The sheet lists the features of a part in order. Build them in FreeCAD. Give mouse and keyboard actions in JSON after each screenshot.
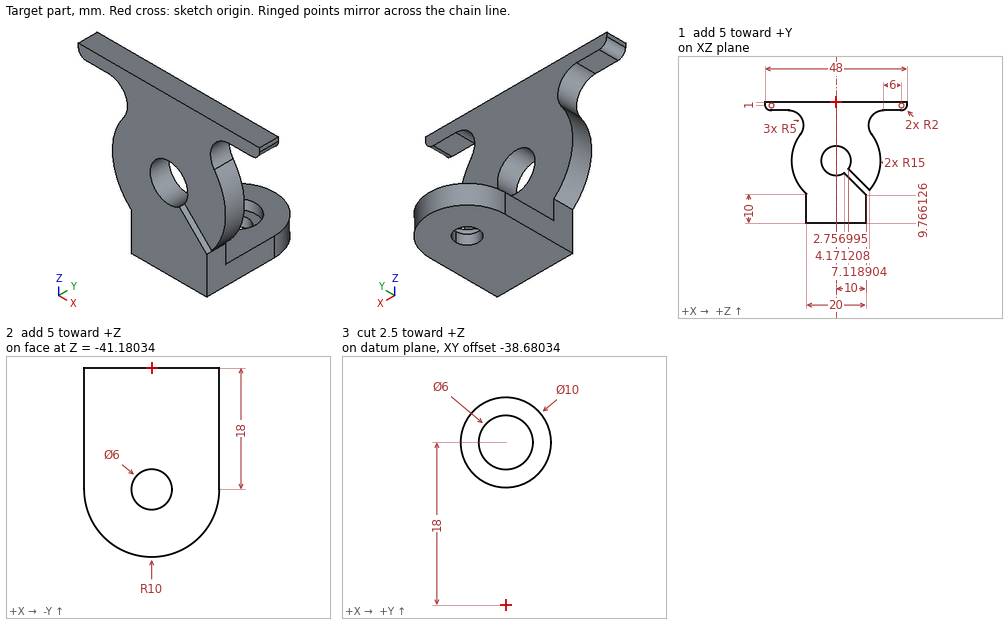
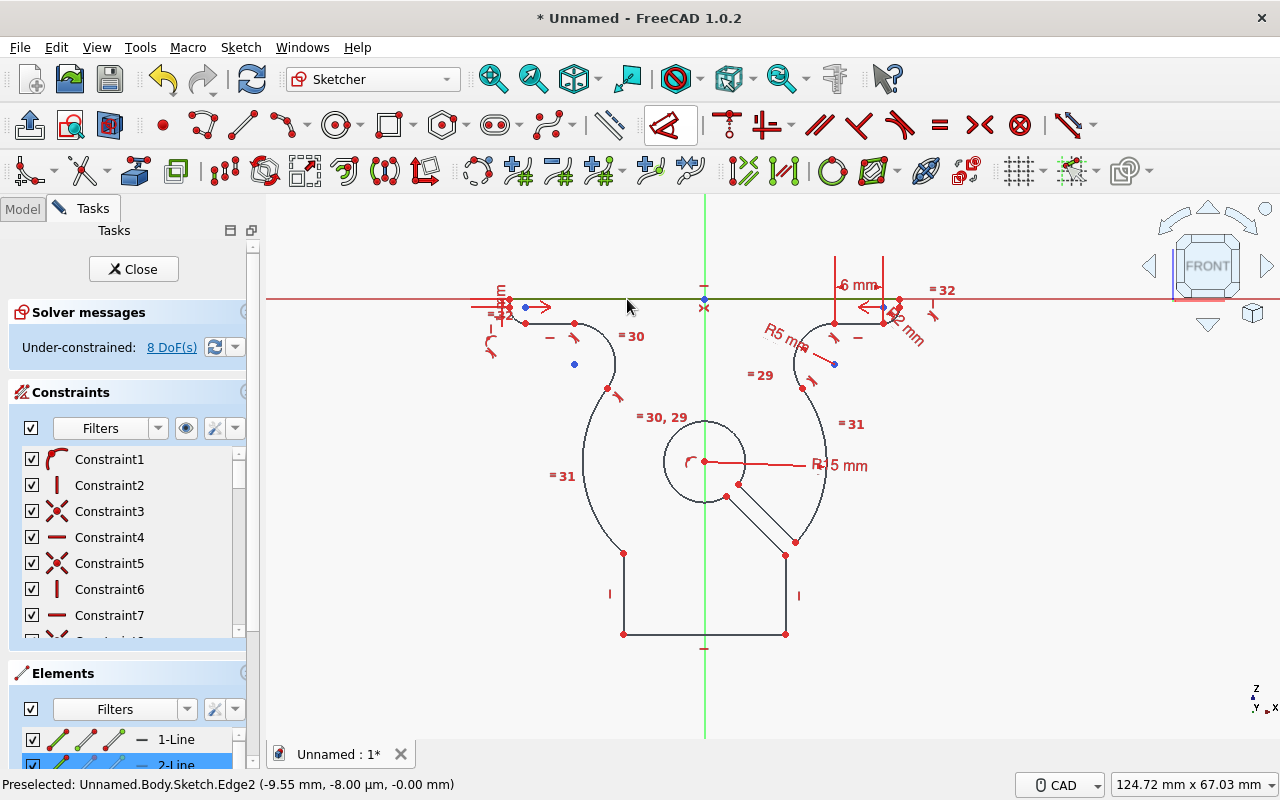
{"action": "key", "text": "l"}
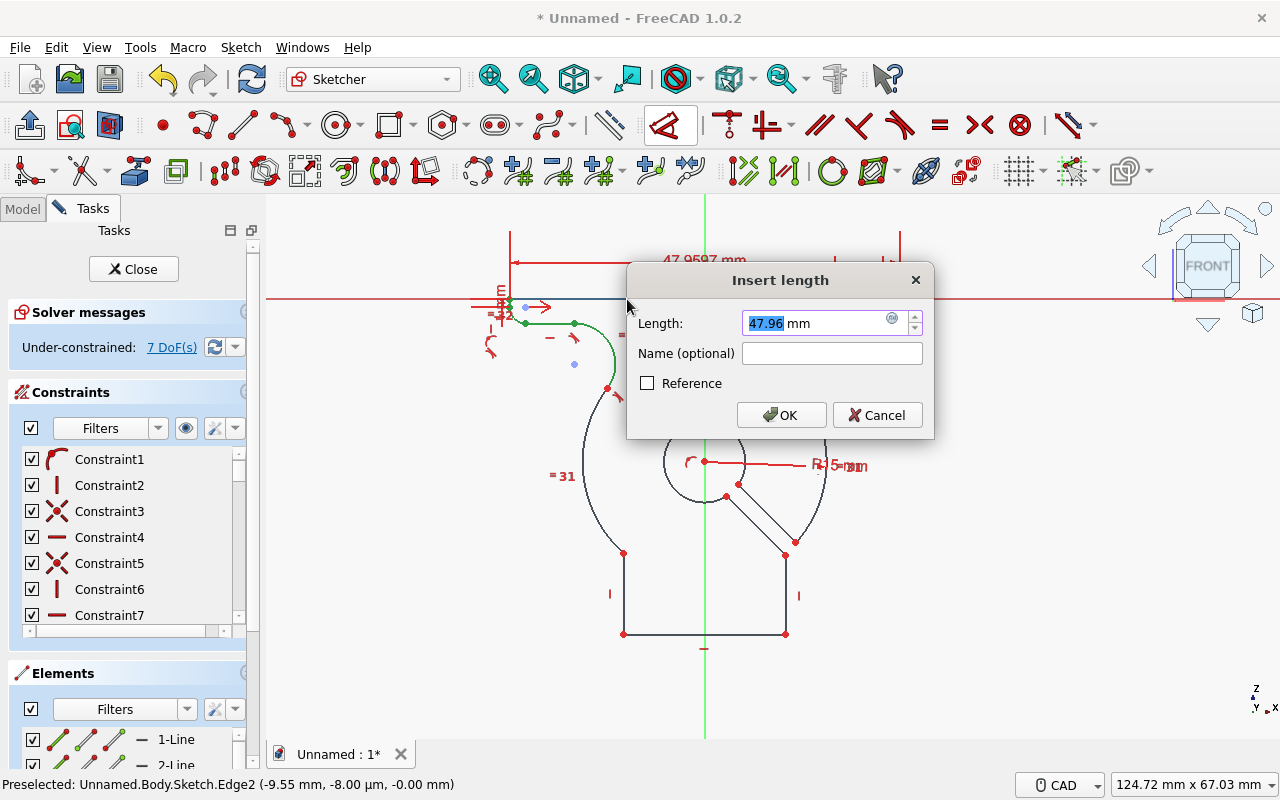
{"action": "type", "text": "48"}
{"action": "key", "text": "Return"}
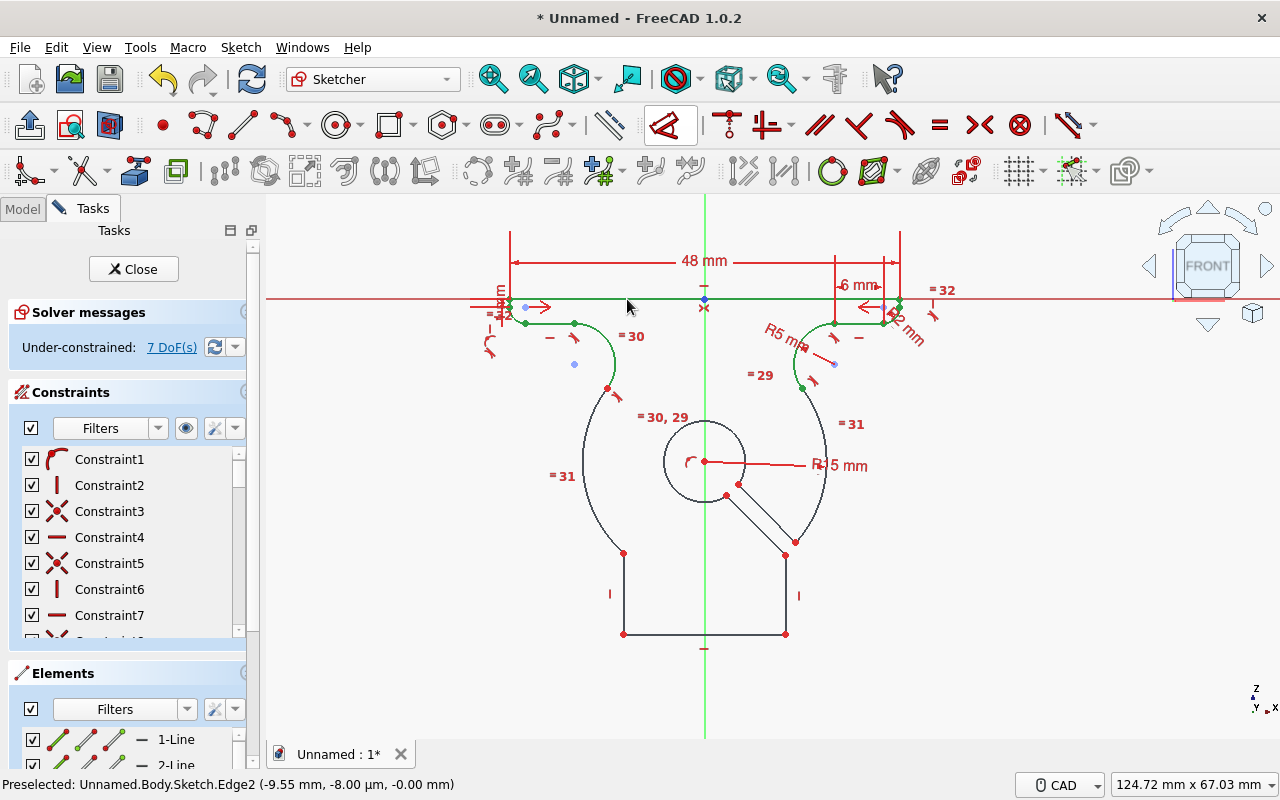
{"action": "left_click", "coordinate": [737, 635]}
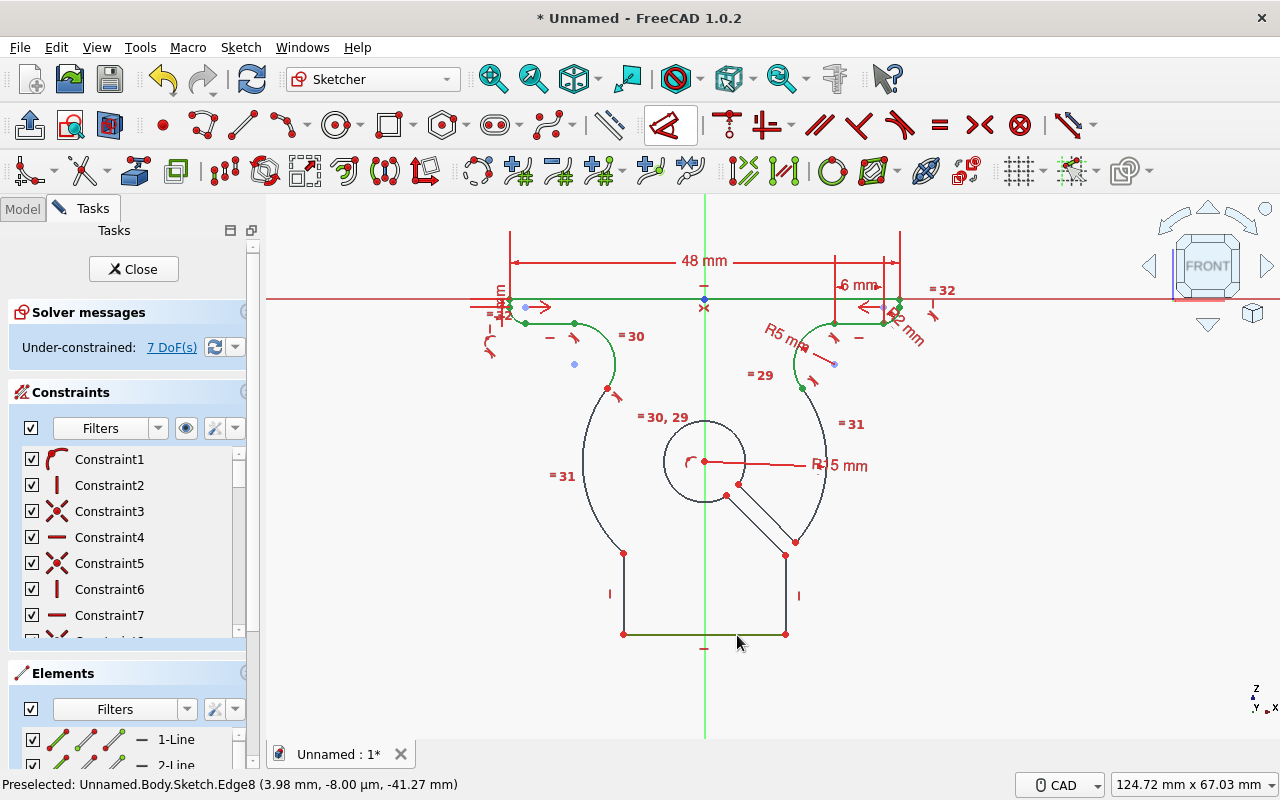
{"action": "key", "text": "l"}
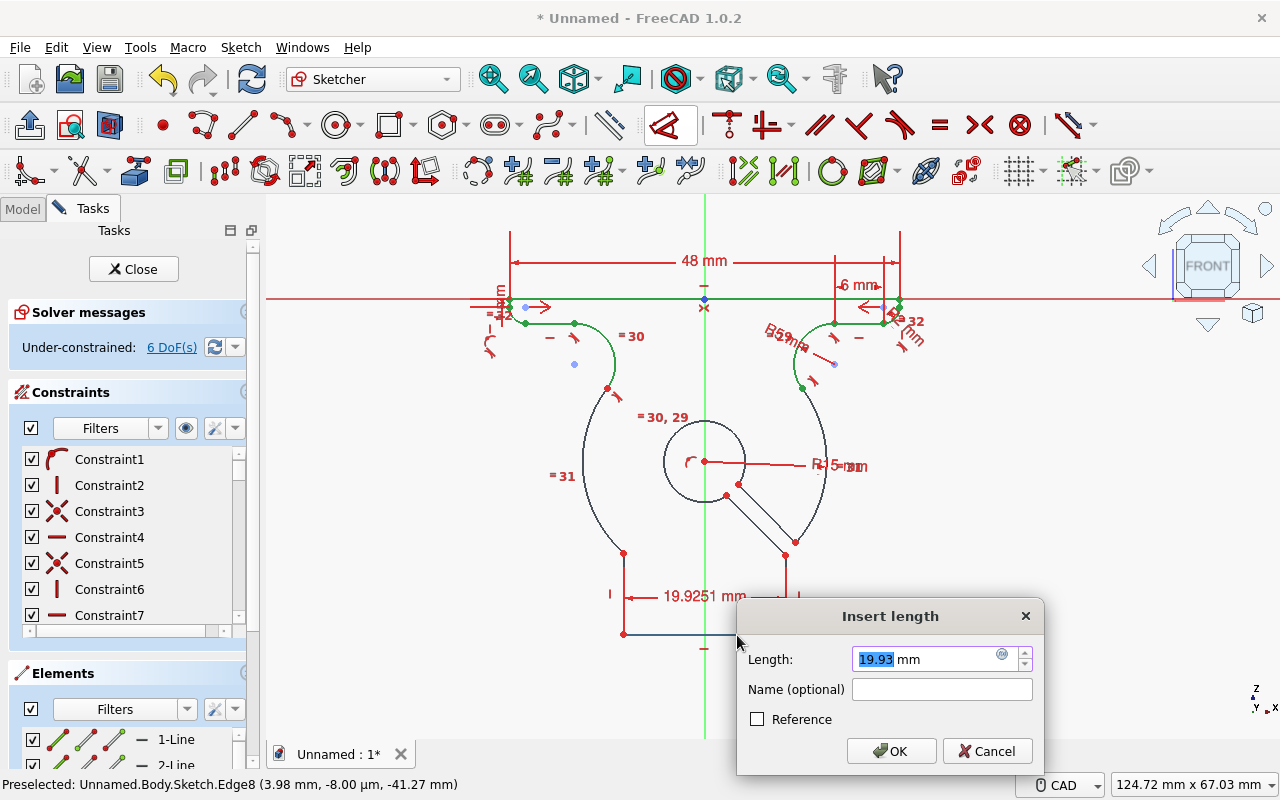
{"action": "type", "text": "20"}
{"action": "key", "text": "Return"}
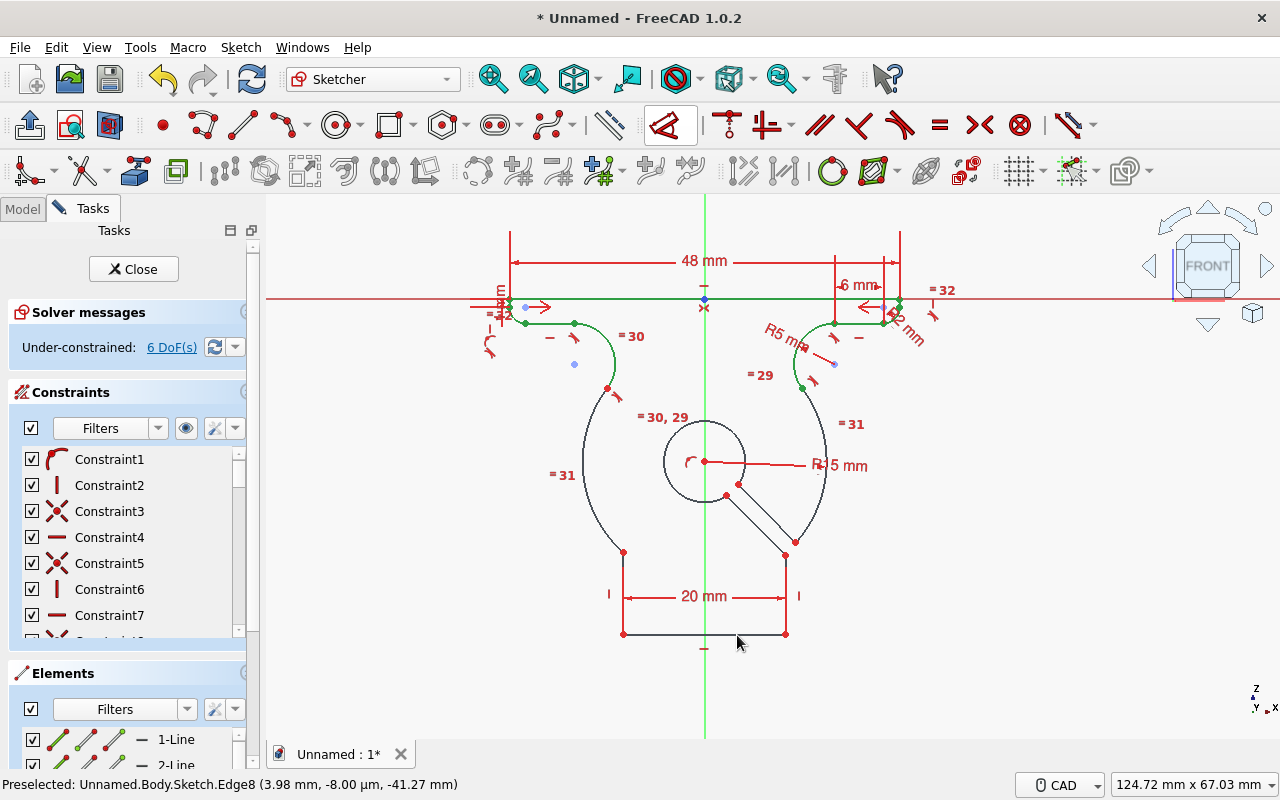
{"action": "left_click", "coordinate": [623, 610]}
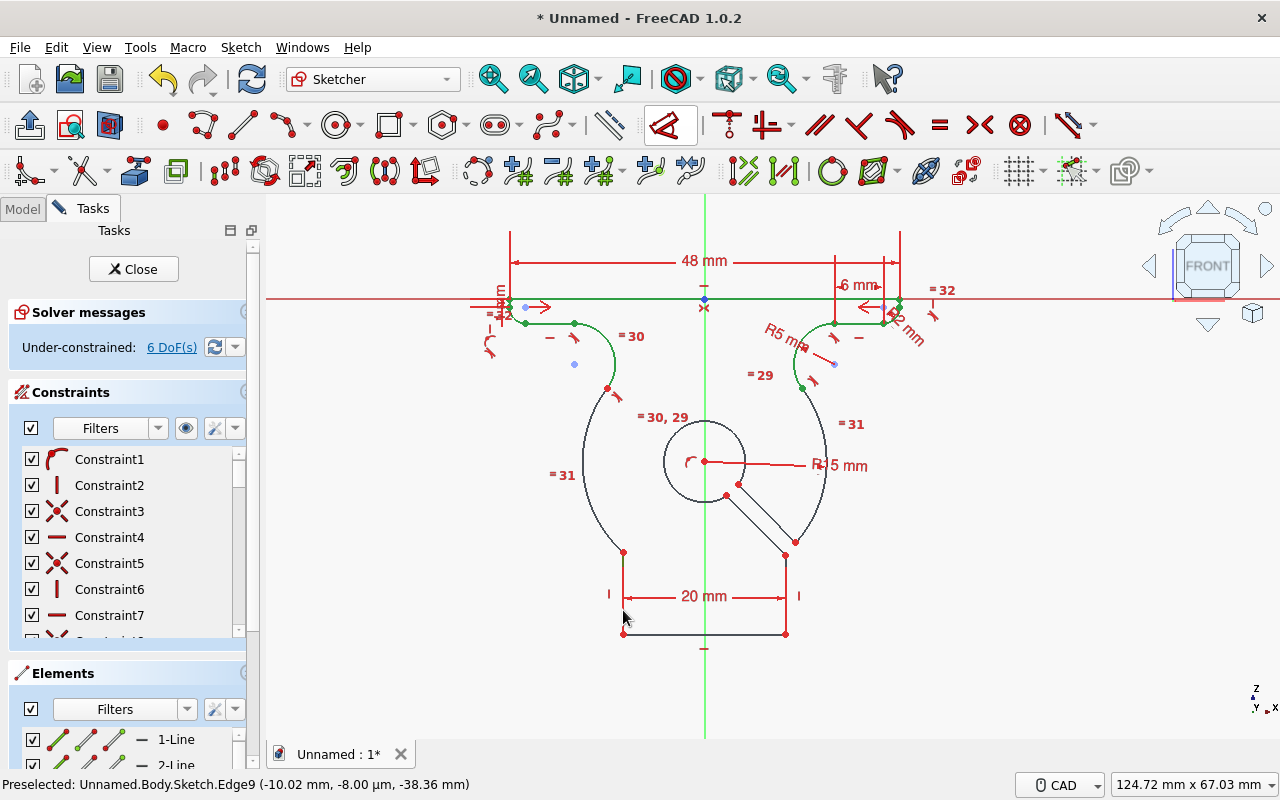
{"action": "key", "text": "i"}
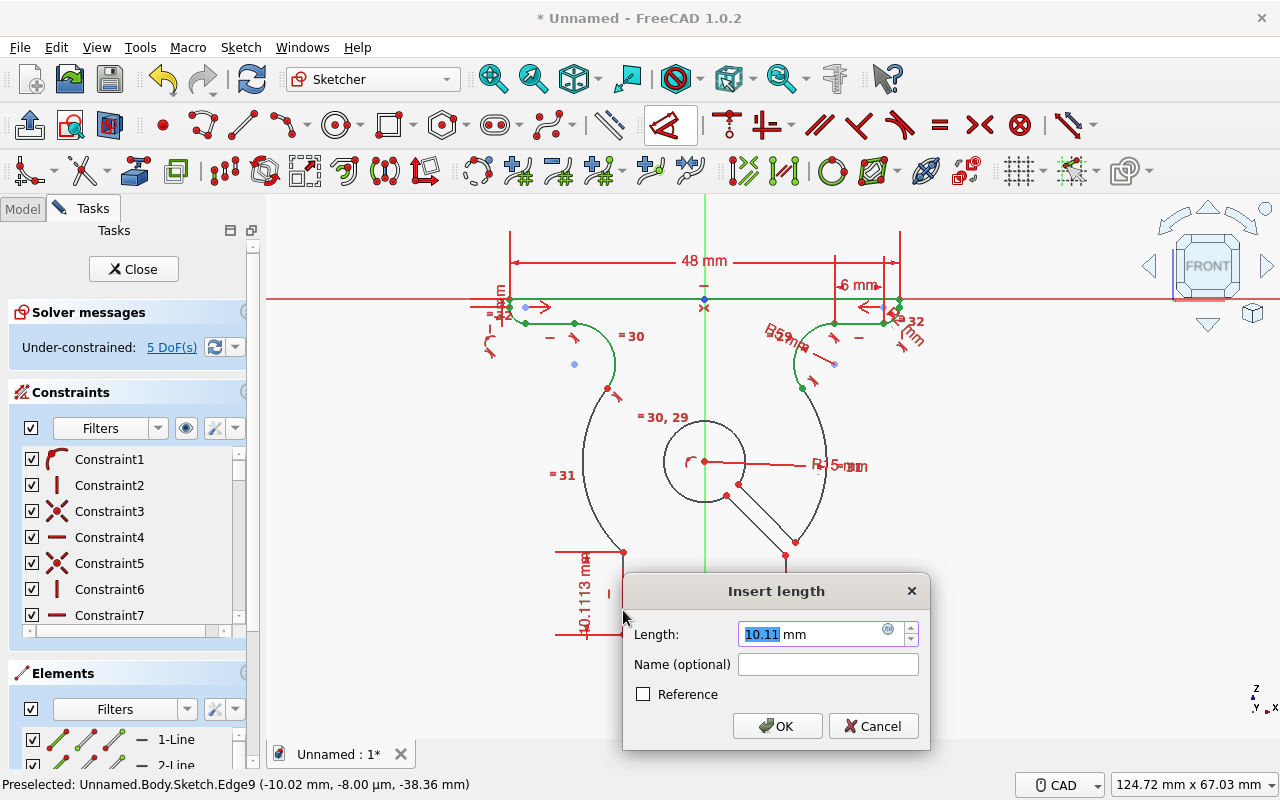
{"action": "type", "text": "10"}
{"action": "key", "text": "Return"}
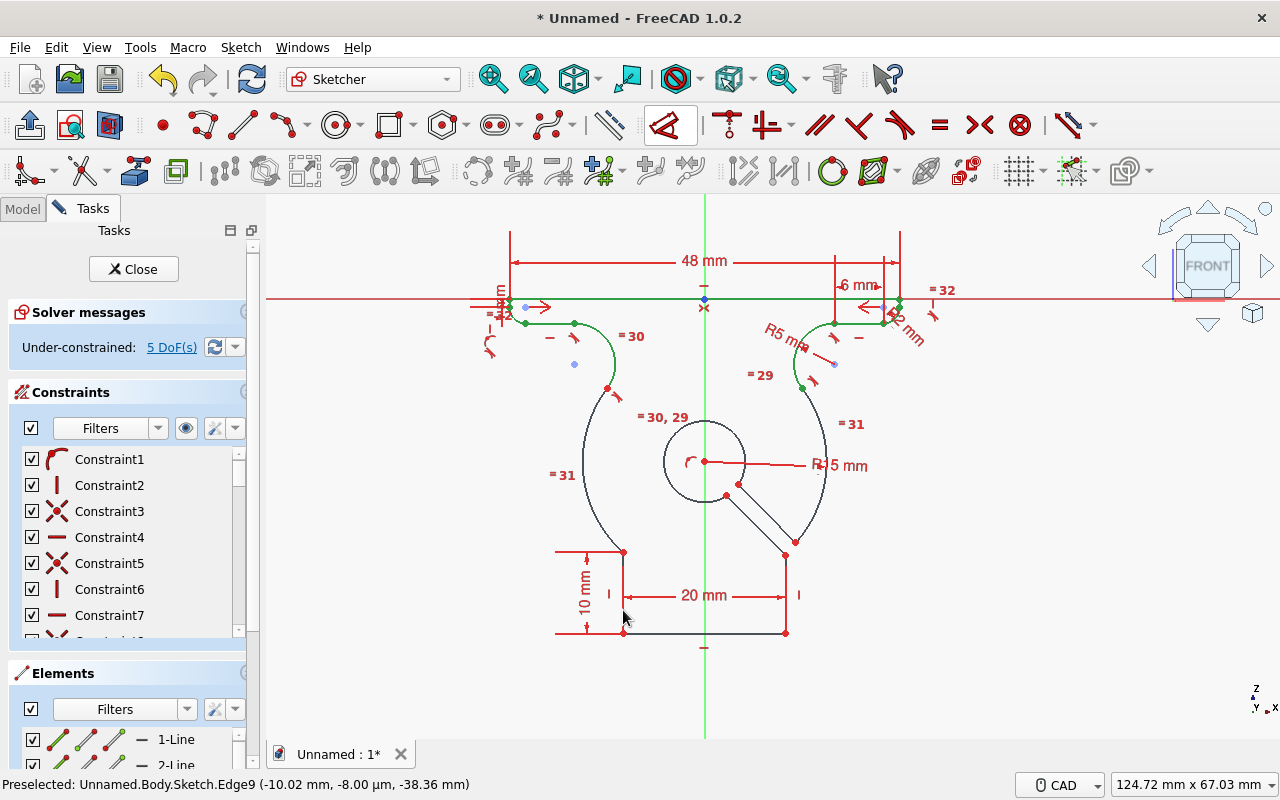
{"action": "left_click", "coordinate": [786, 556]}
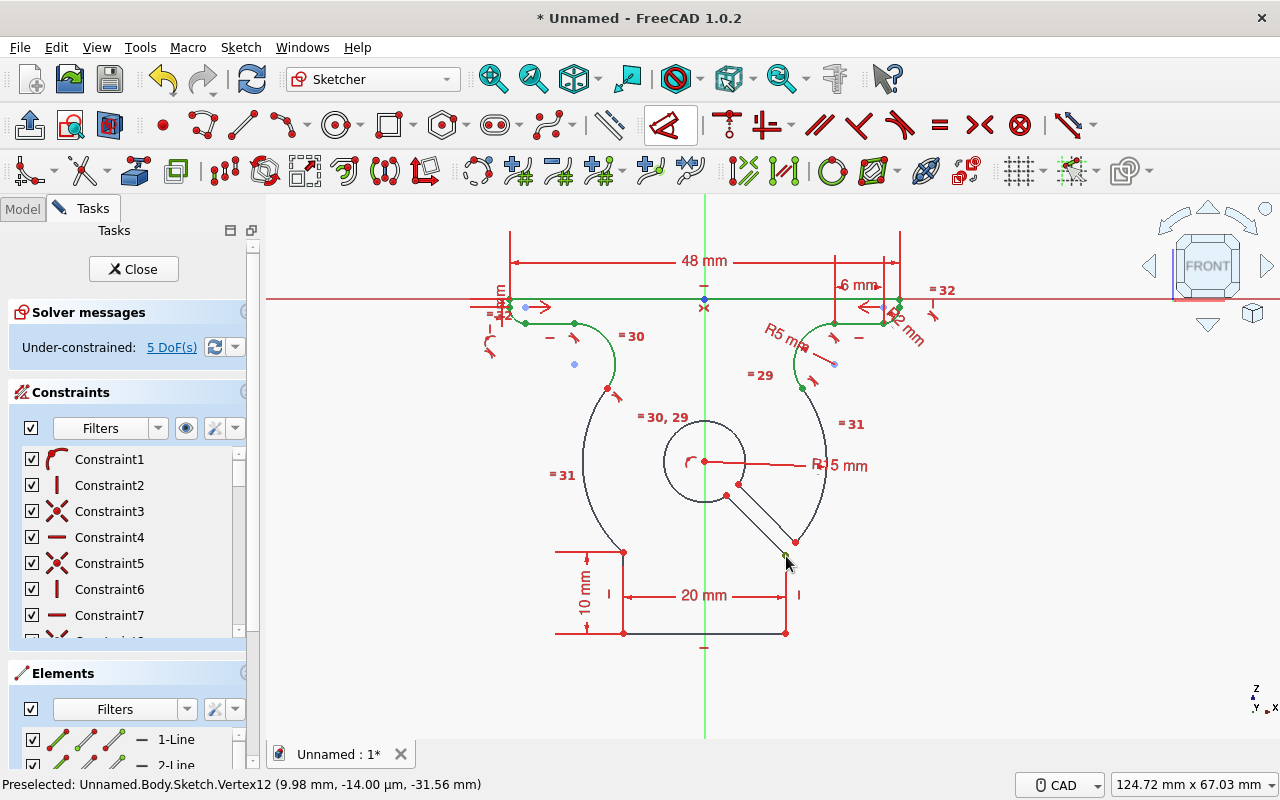
{"action": "key", "text": "l"}